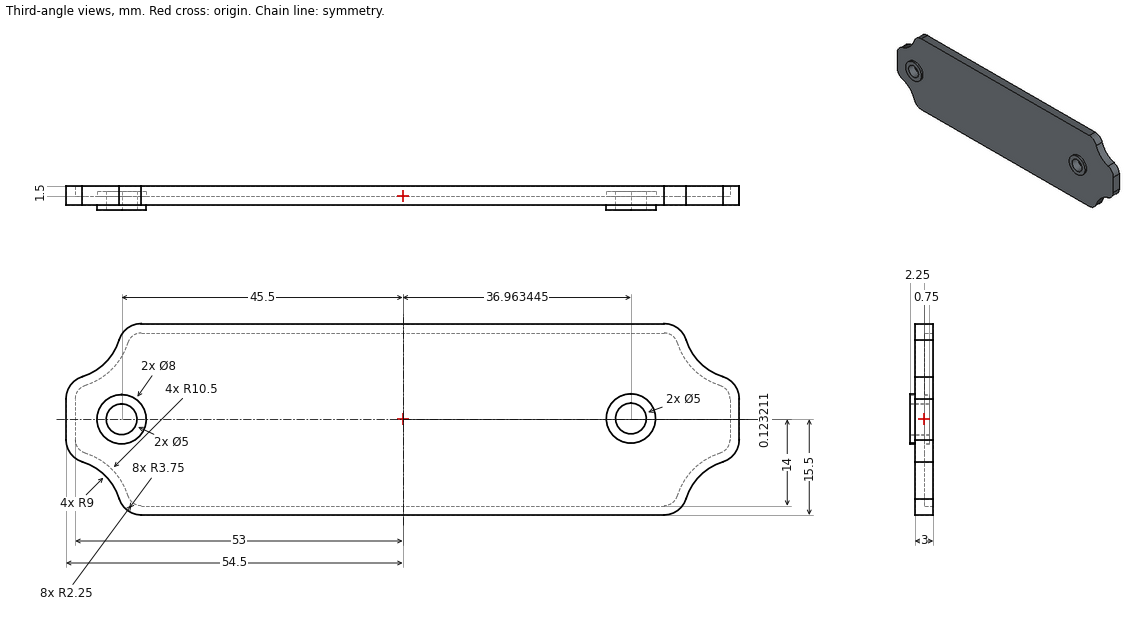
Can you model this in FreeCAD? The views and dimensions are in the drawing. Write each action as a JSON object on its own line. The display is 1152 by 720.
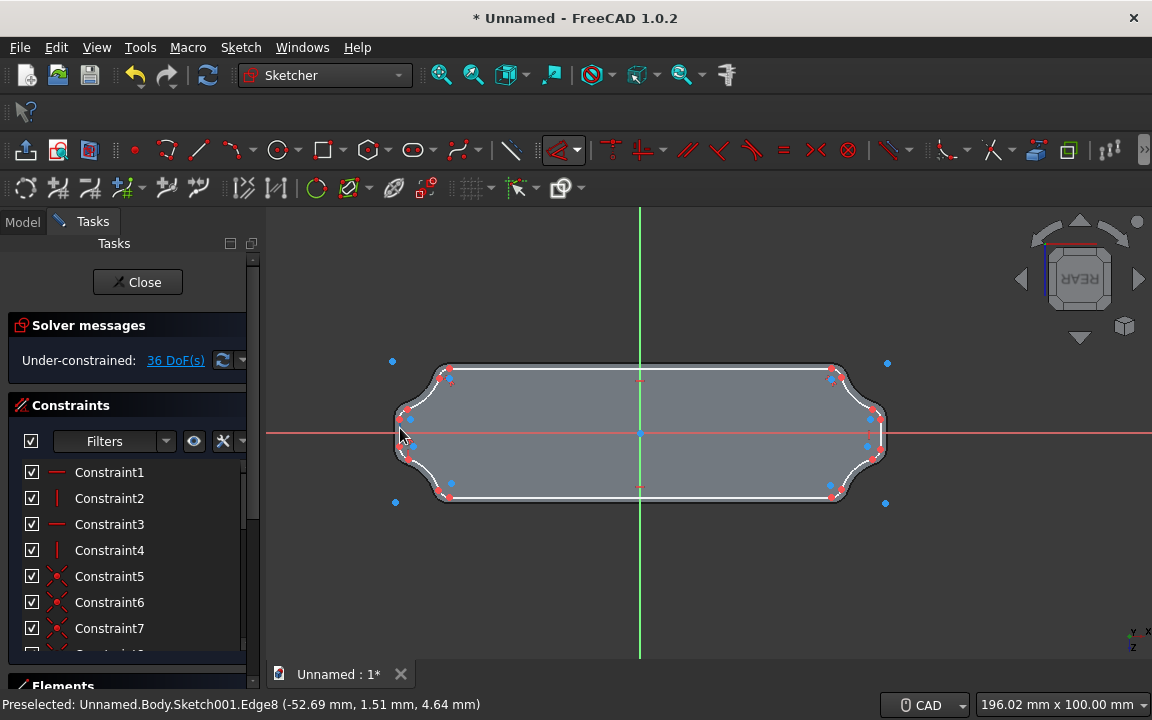
{"action": "left_click", "coordinate": [564, 498]}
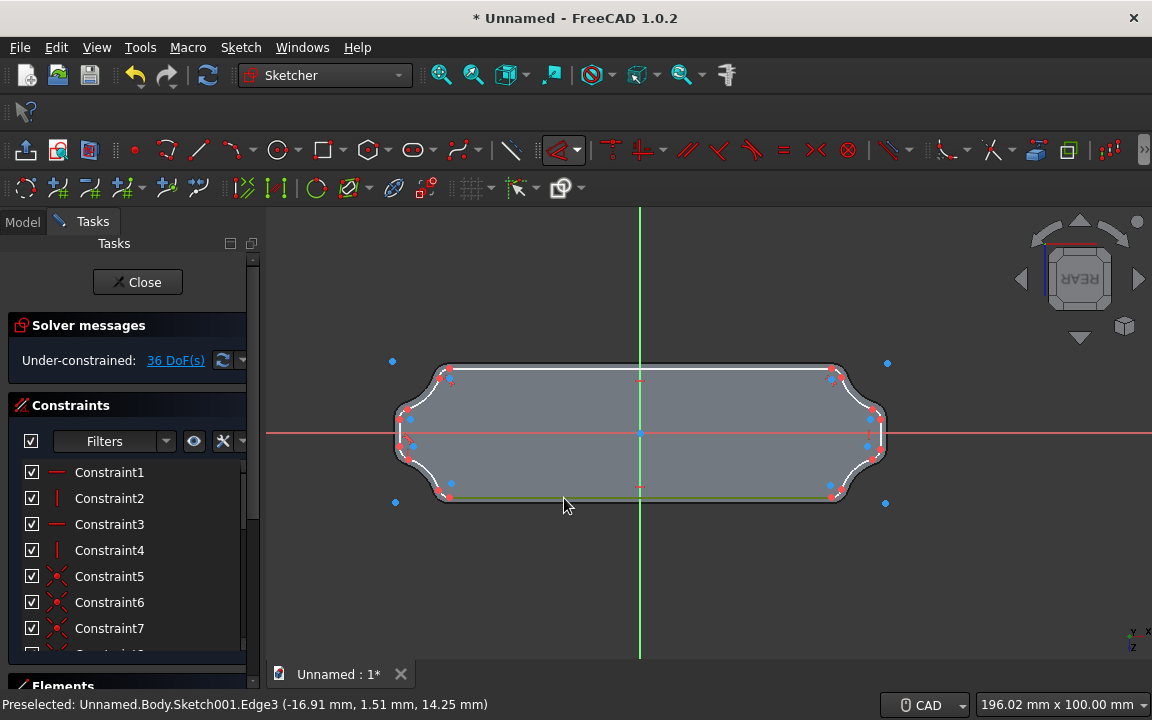
{"action": "scroll", "coordinate": [443, 495], "scroll_direction": "up", "scroll_amount": 4}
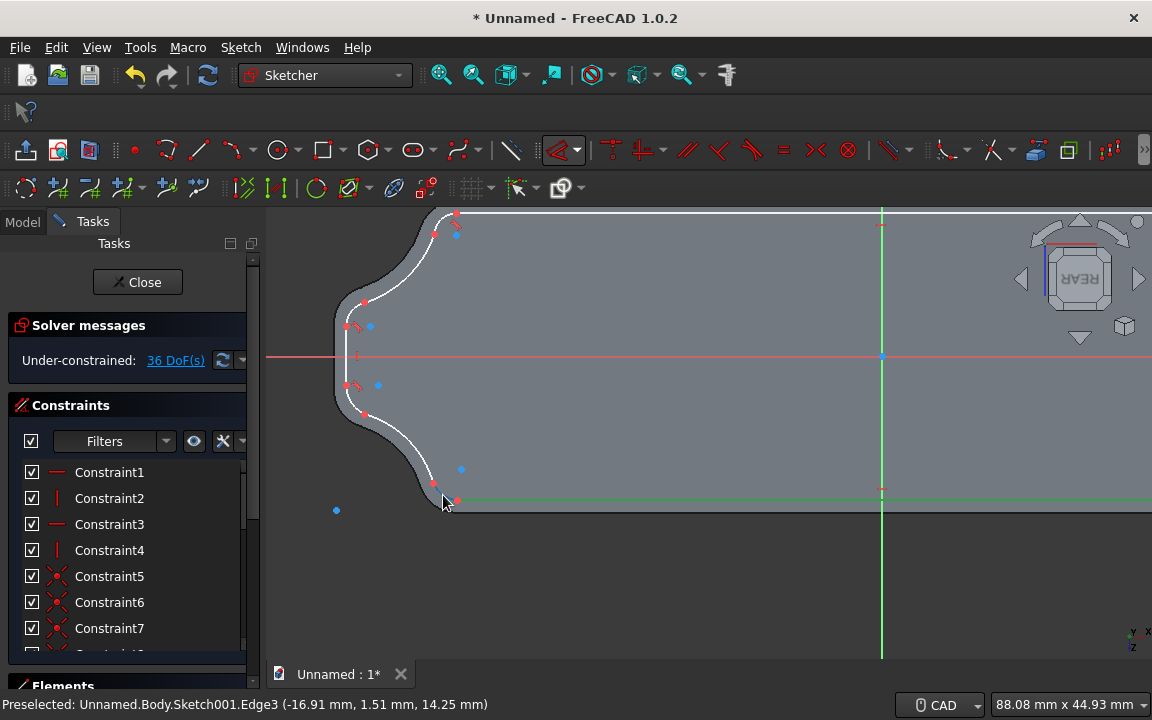
{"action": "left_click", "coordinate": [443, 495]}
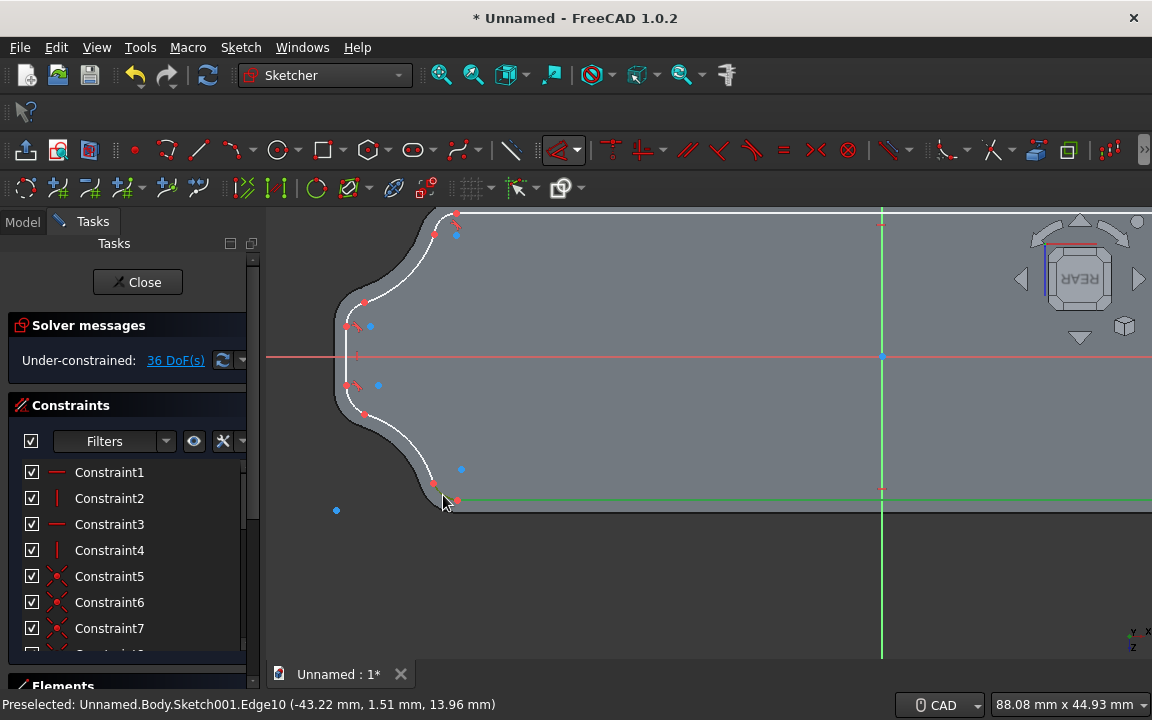
{"action": "left_click", "coordinate": [752, 150]}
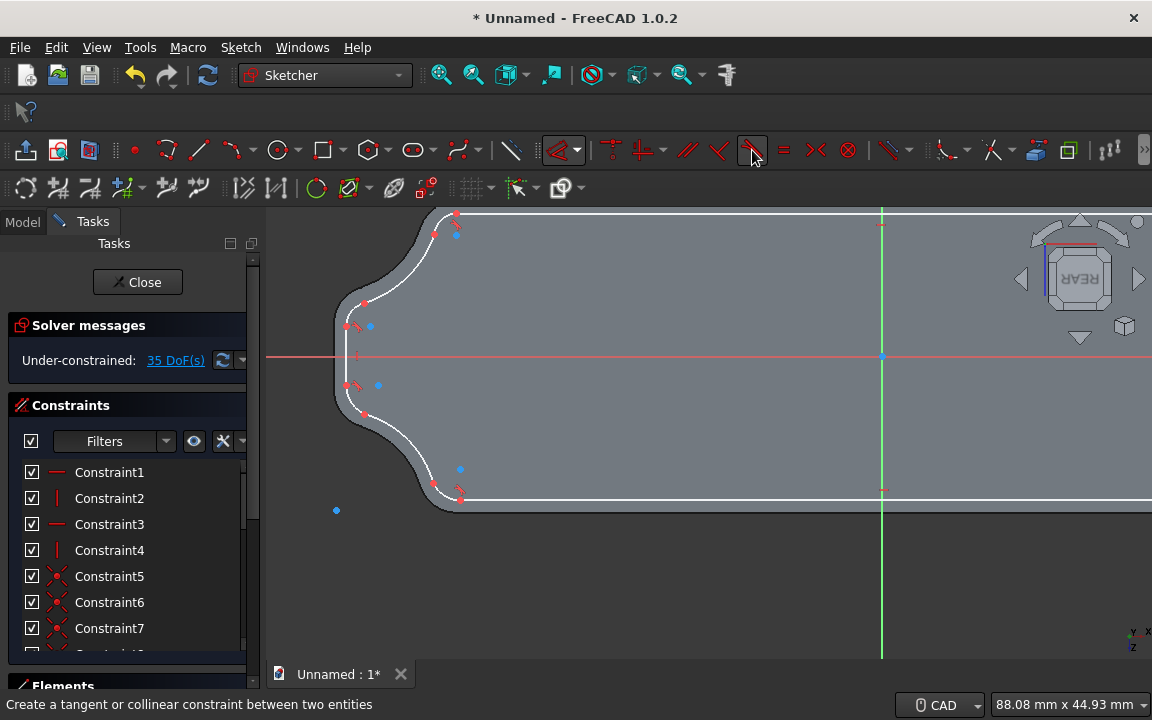
{"action": "left_click", "coordinate": [715, 500]}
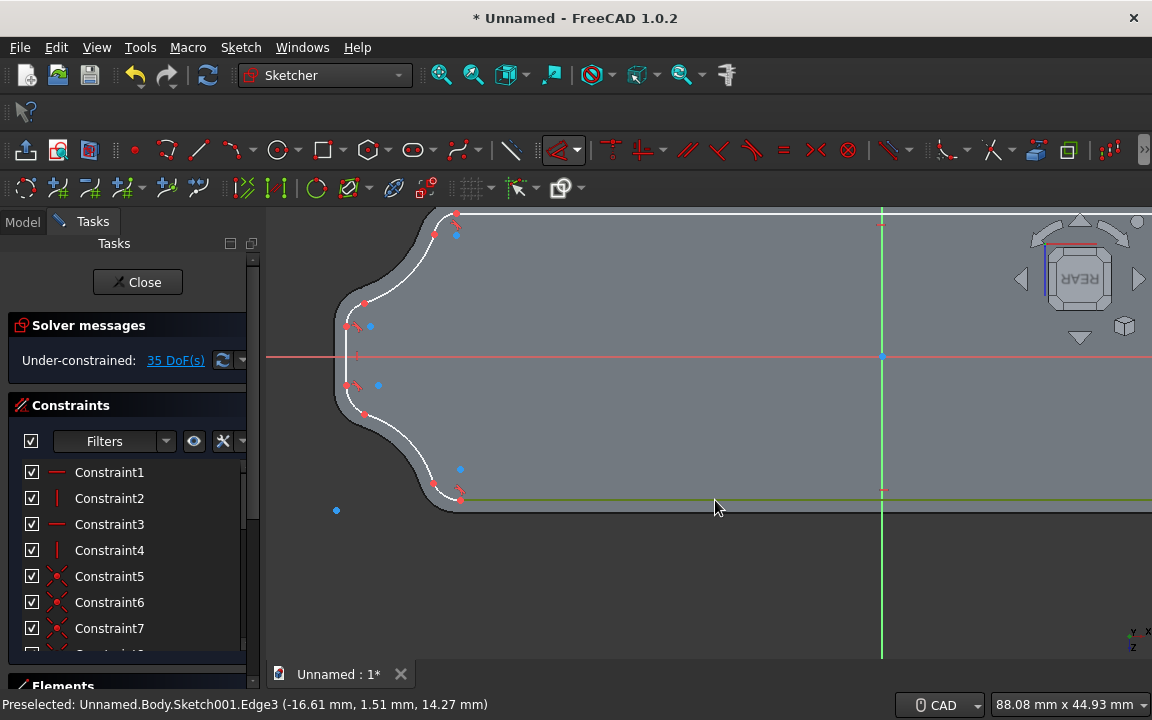
{"action": "scroll", "coordinate": [443, 495], "scroll_direction": "down", "scroll_amount": 4}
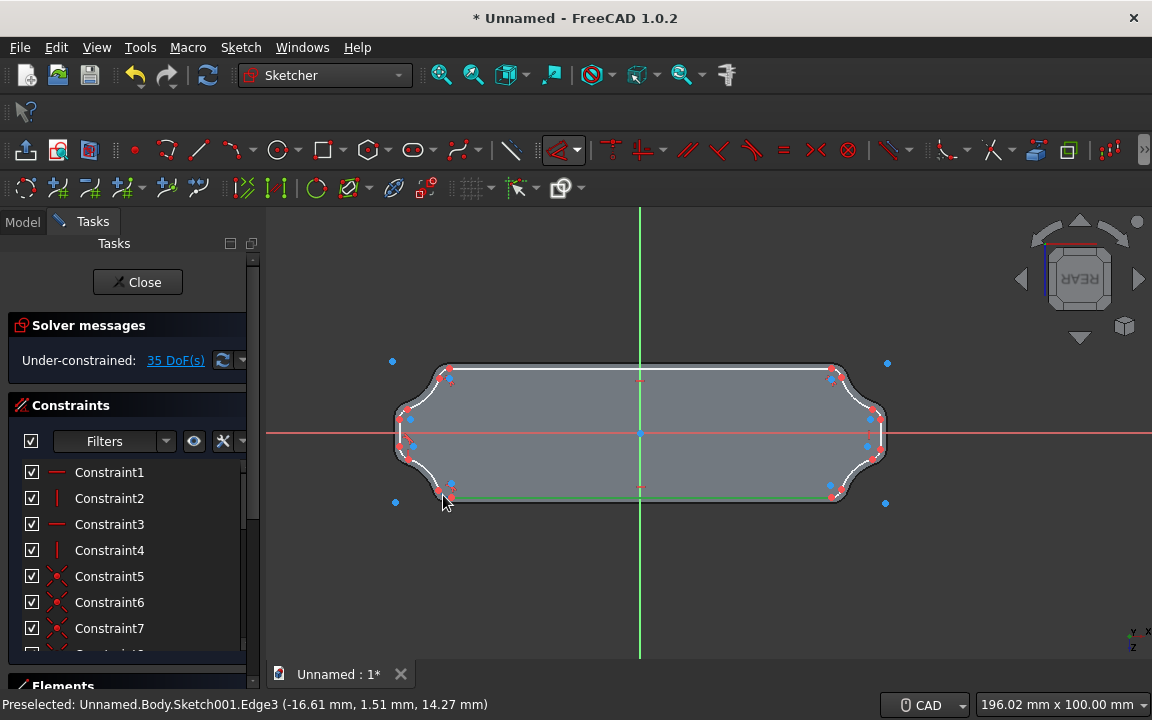
{"action": "scroll", "coordinate": [835, 497], "scroll_direction": "up", "scroll_amount": 7}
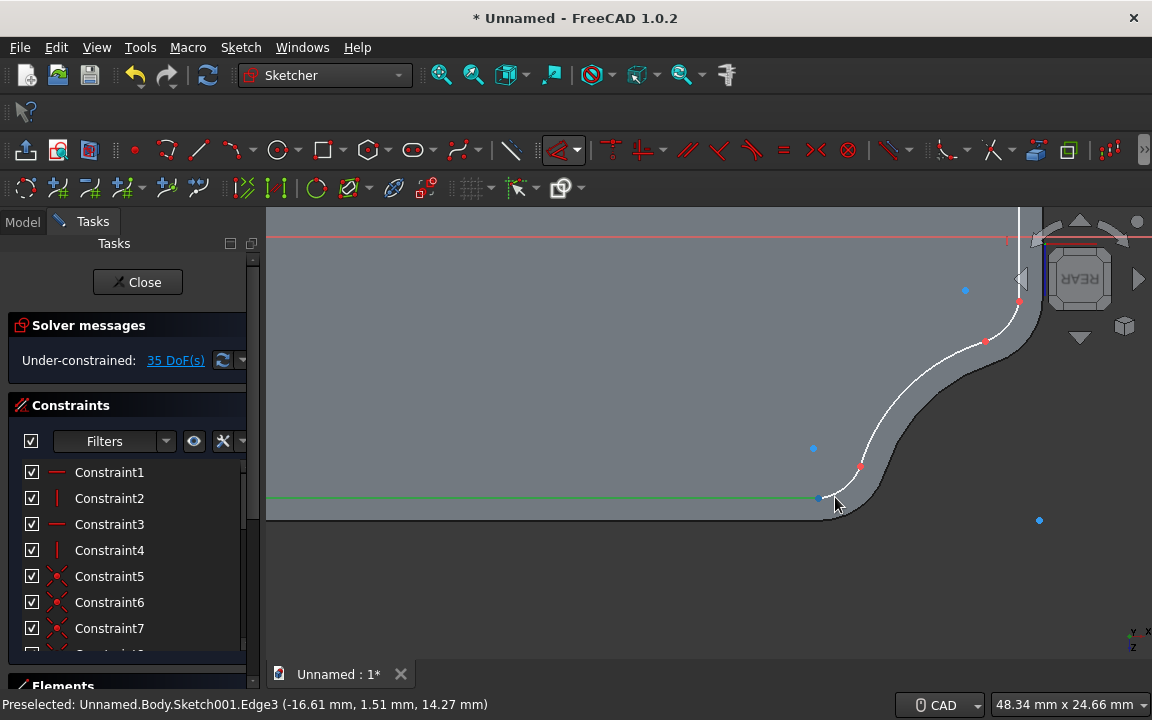
{"action": "left_click", "coordinate": [834, 494]}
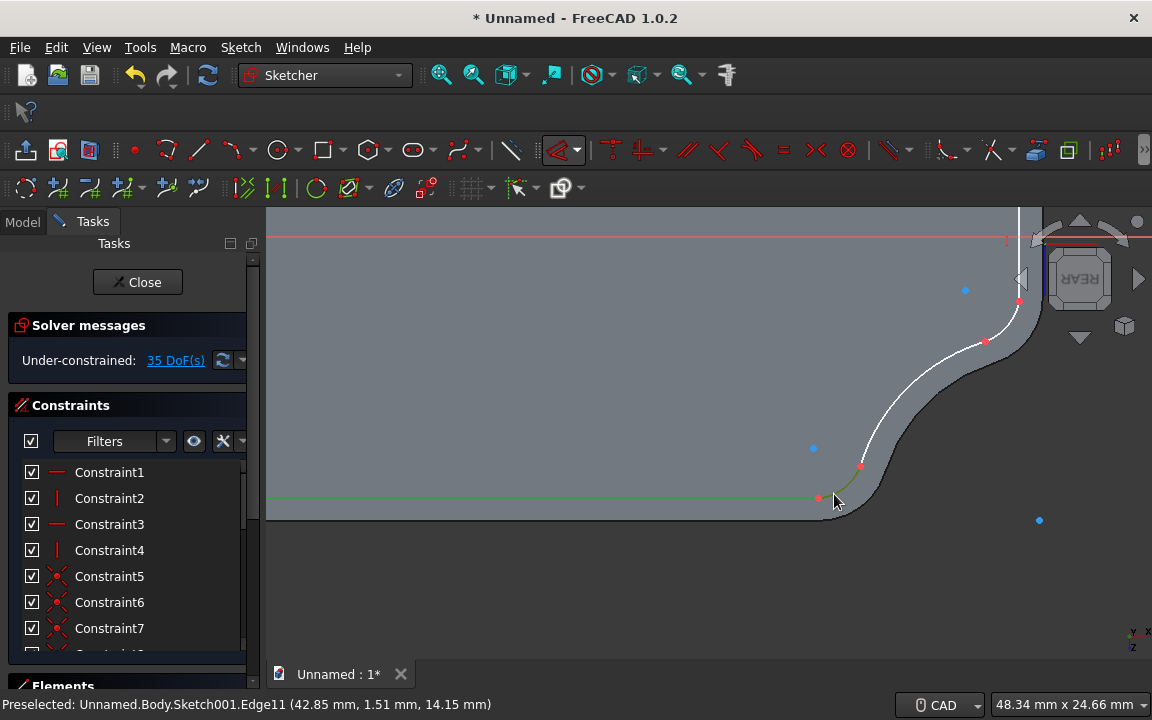
{"action": "left_click", "coordinate": [752, 150]}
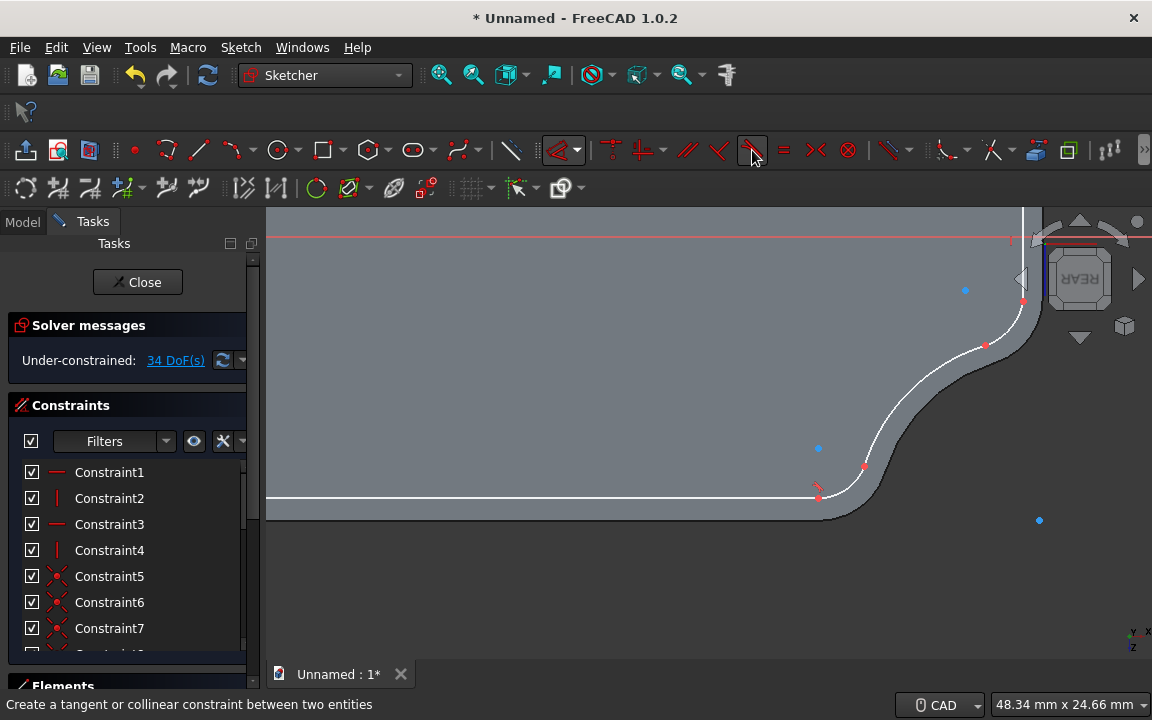
{"action": "scroll", "coordinate": [836, 497], "scroll_direction": "down", "scroll_amount": 7}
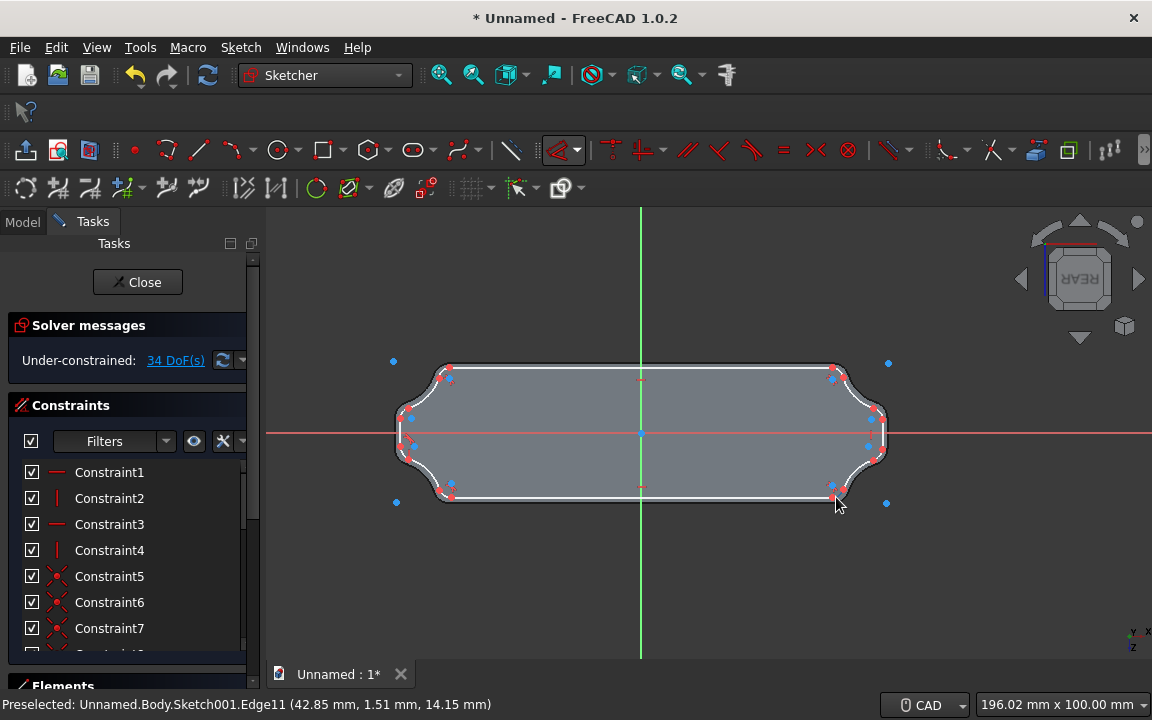
{"action": "scroll", "coordinate": [883, 440], "scroll_direction": "up", "scroll_amount": 4}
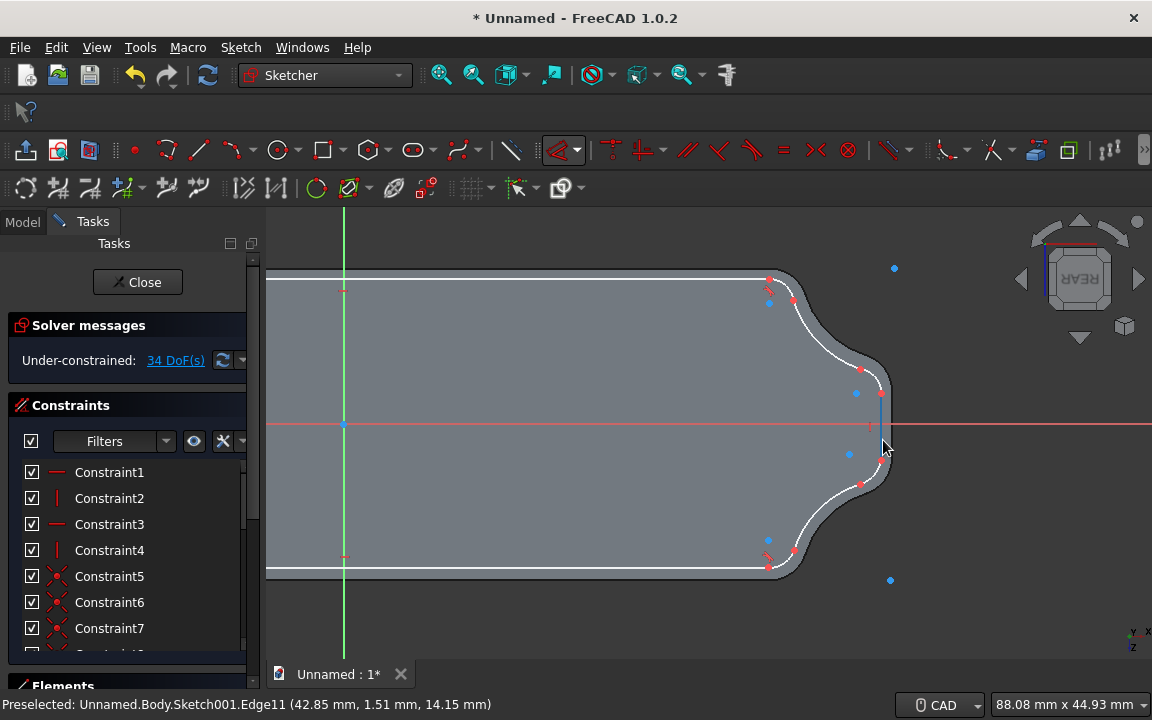
{"action": "left_click", "coordinate": [881, 440]}